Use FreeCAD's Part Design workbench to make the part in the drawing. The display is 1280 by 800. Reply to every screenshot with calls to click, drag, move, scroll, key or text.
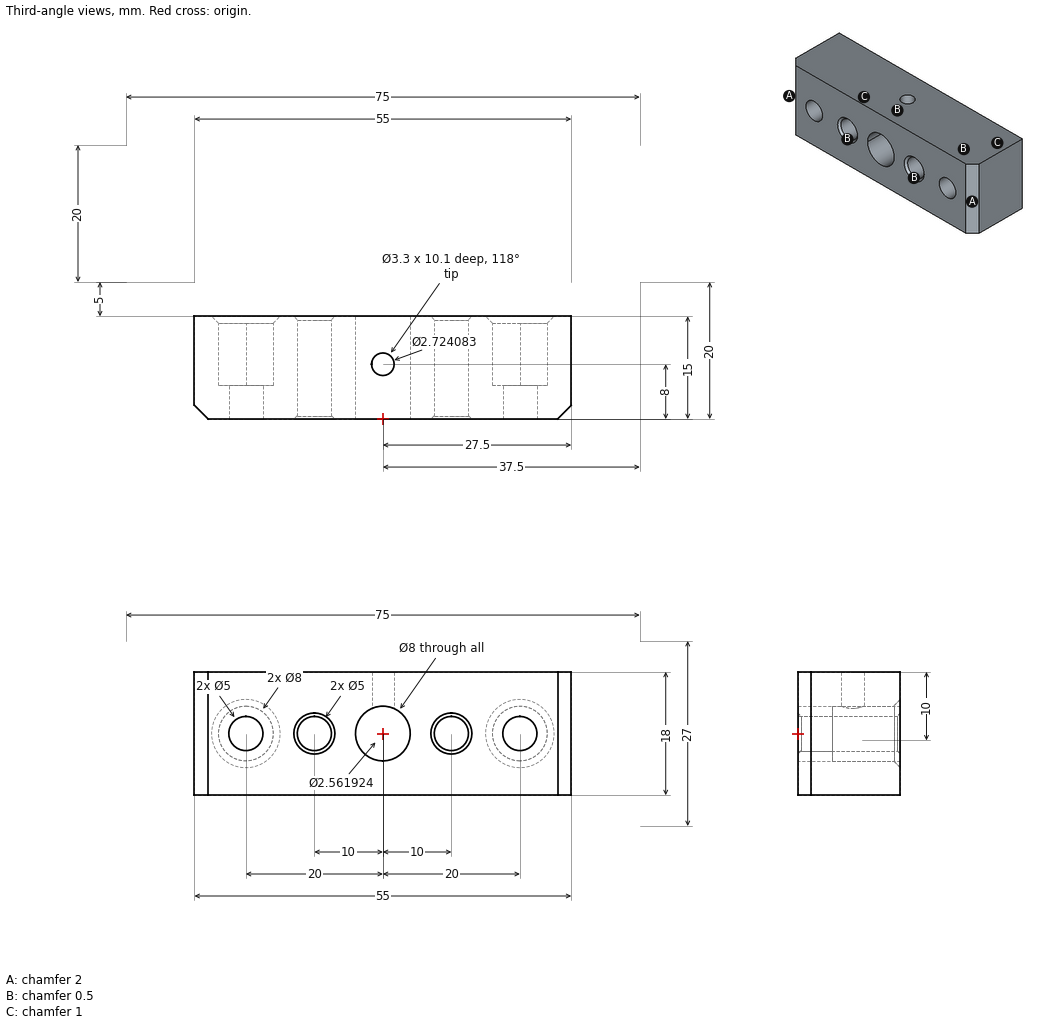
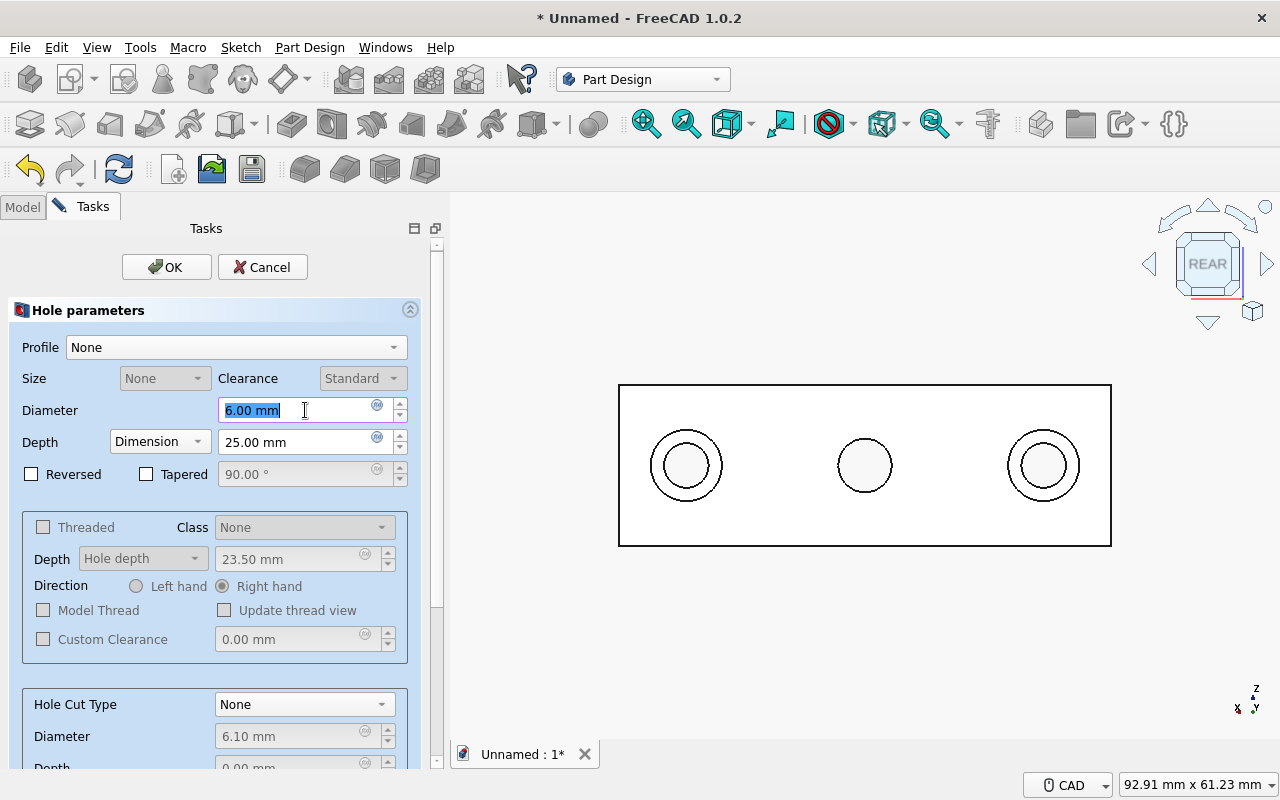
text(8)
key(Tab)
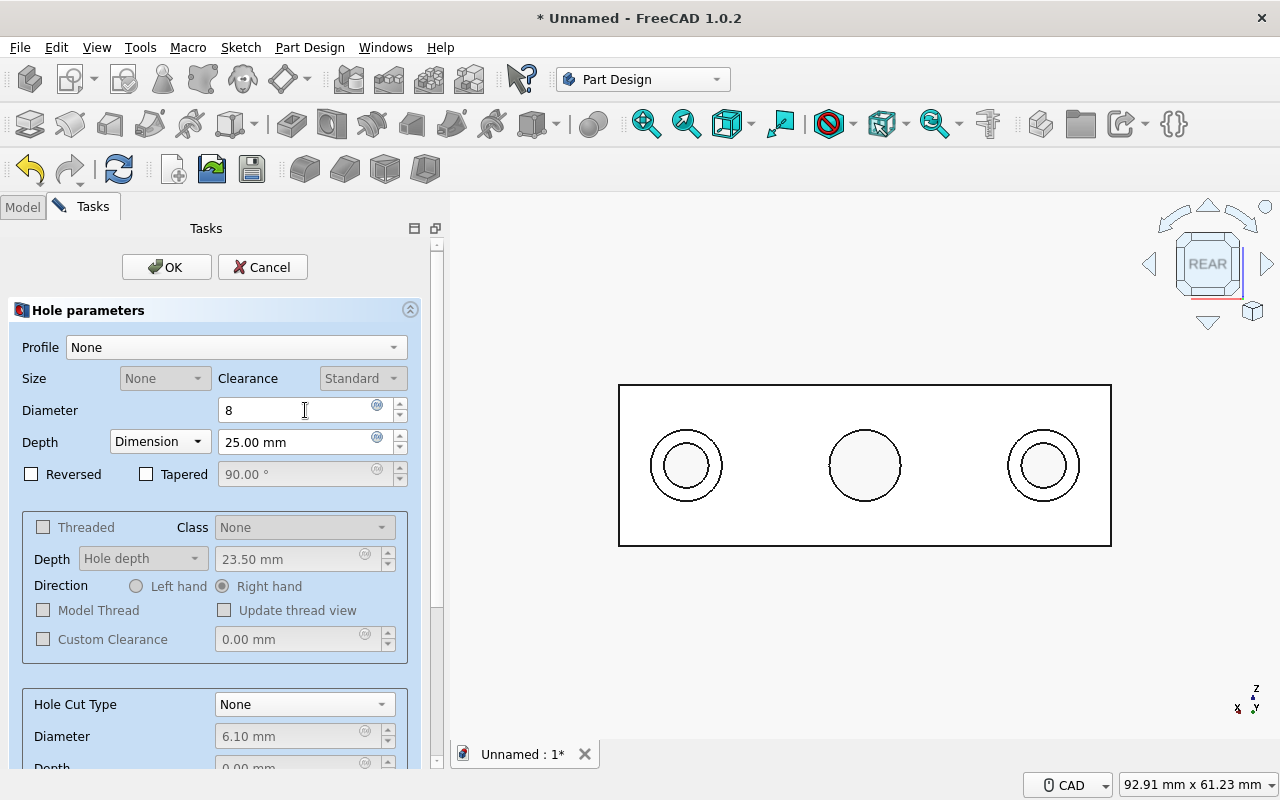
click(161, 442)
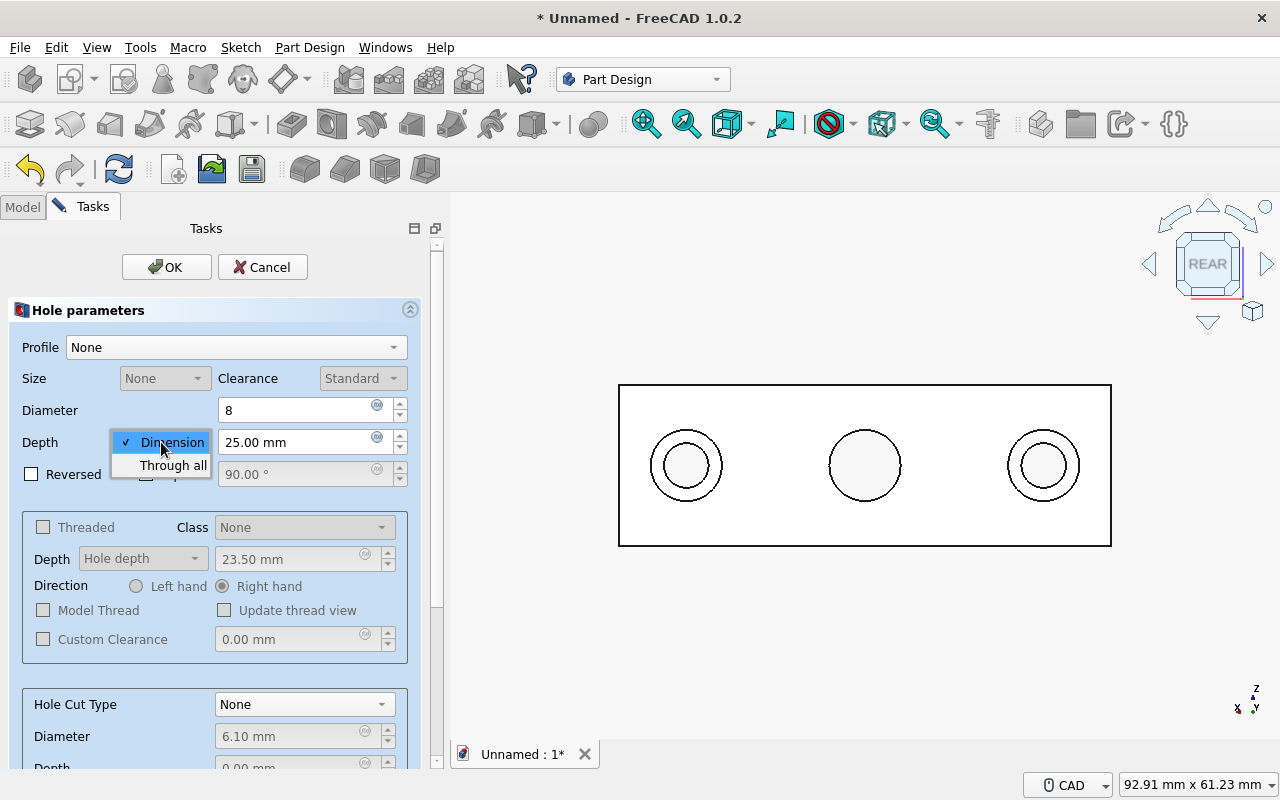
click(160, 466)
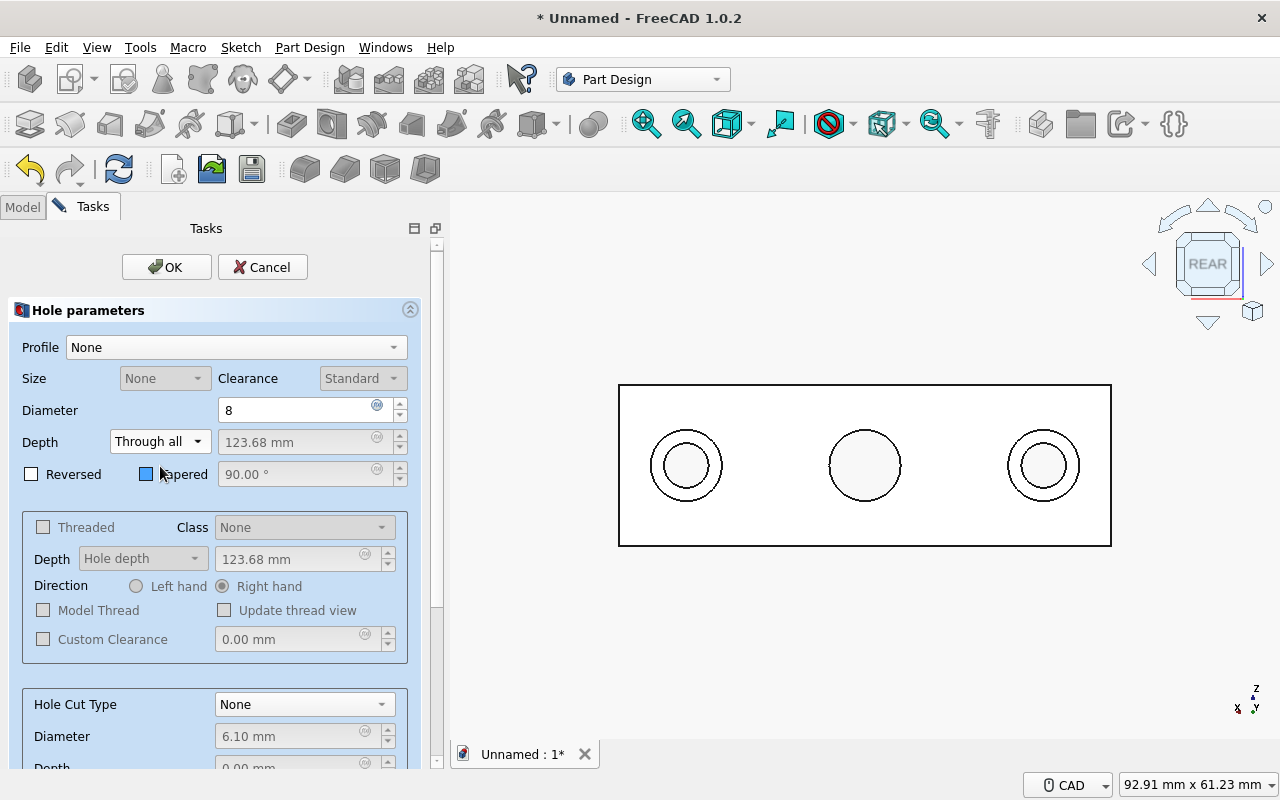
click(167, 267)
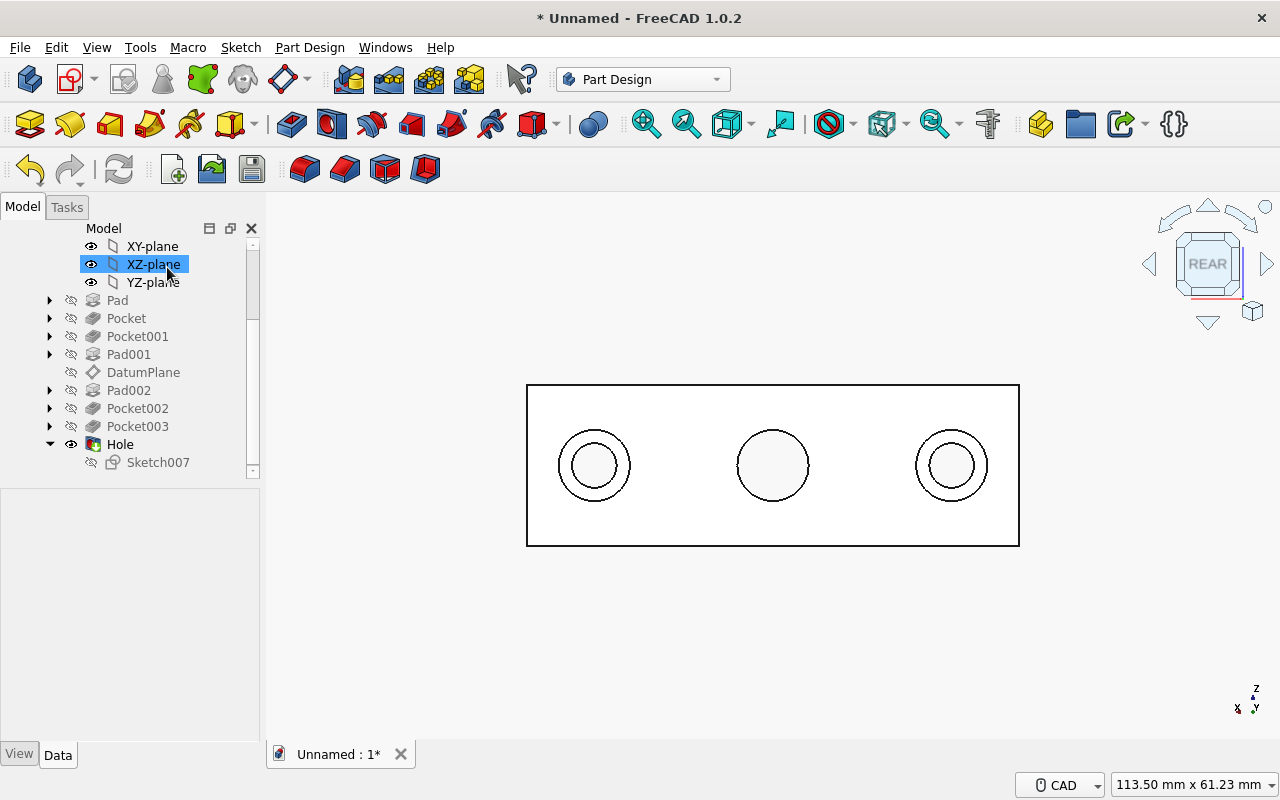
key(0)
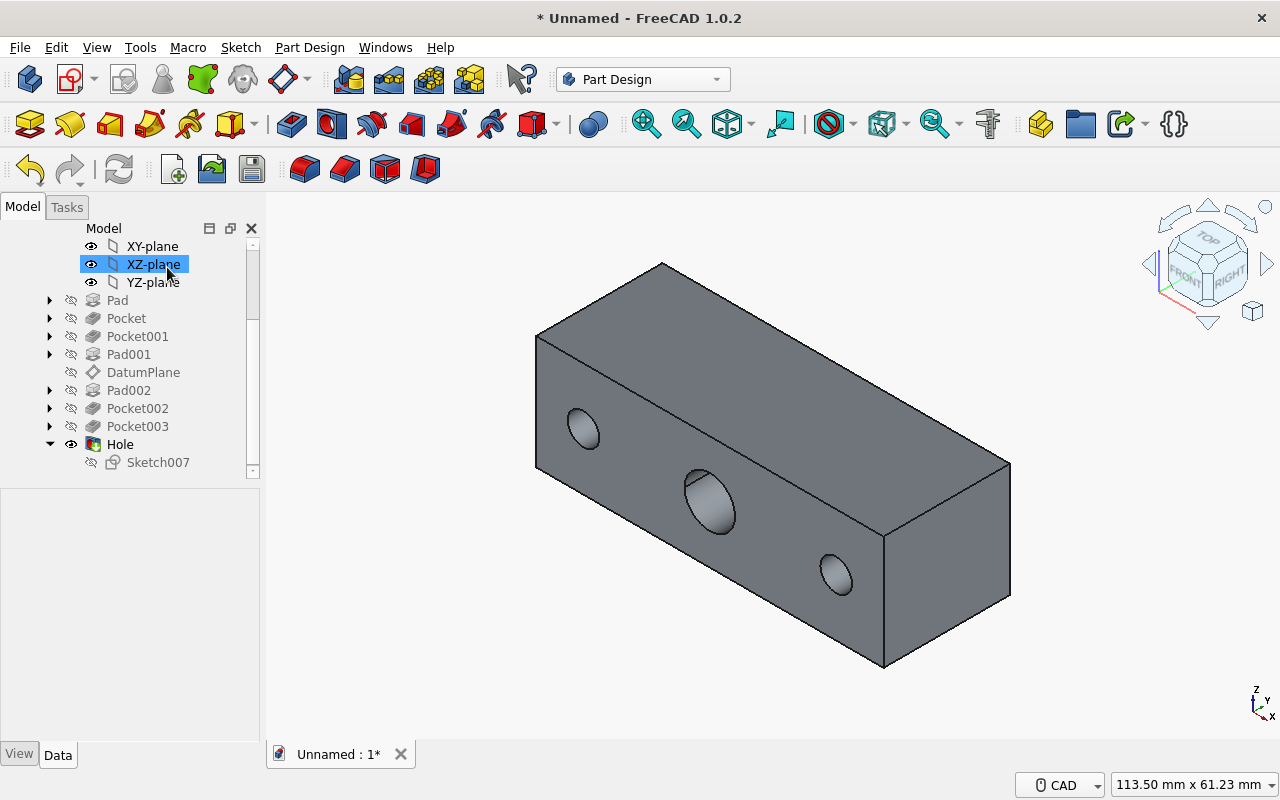
click(884, 601)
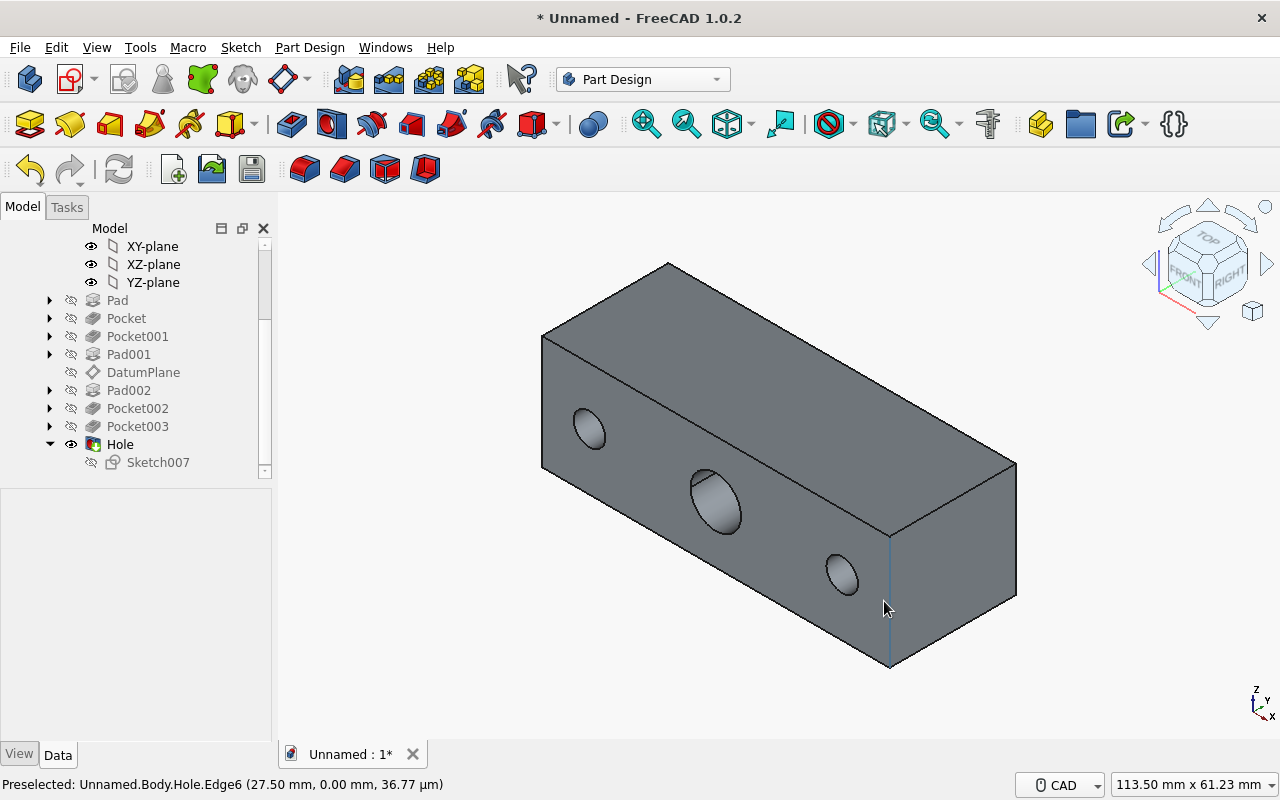
key(2)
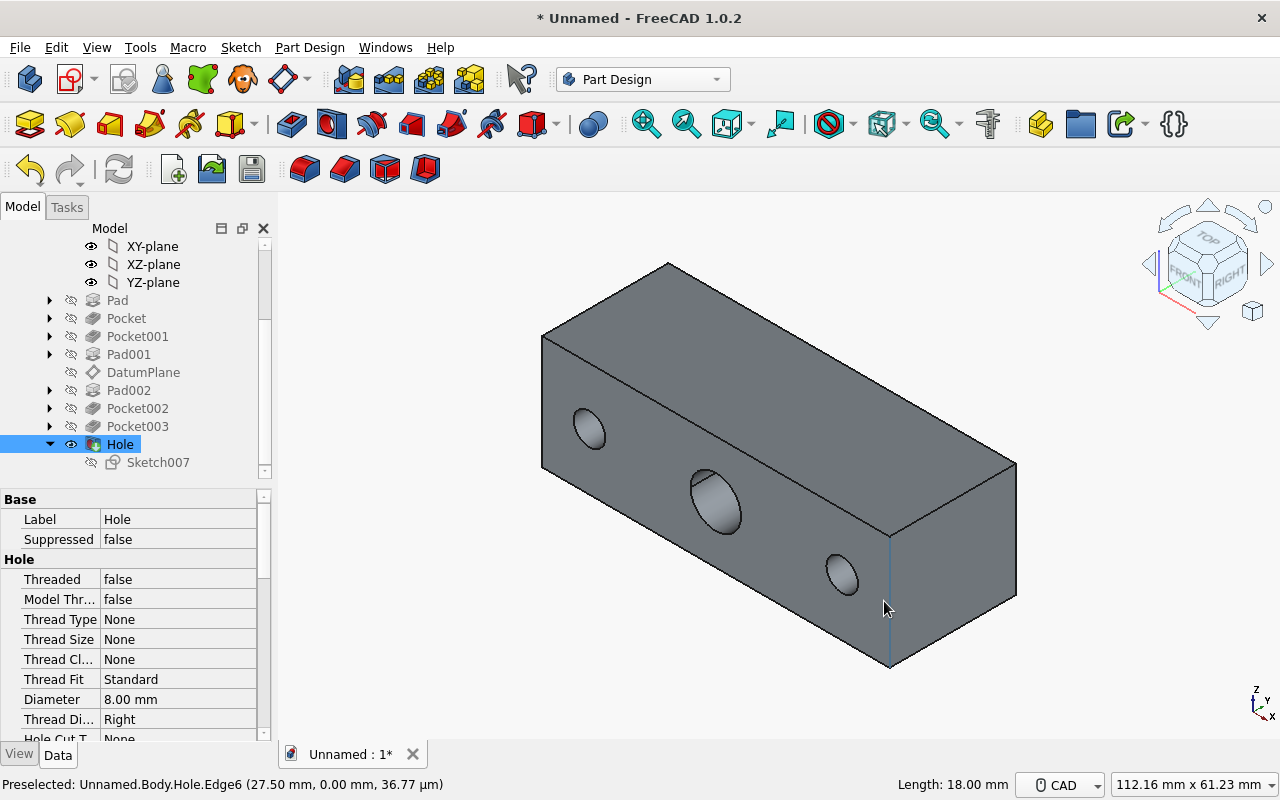
key(1)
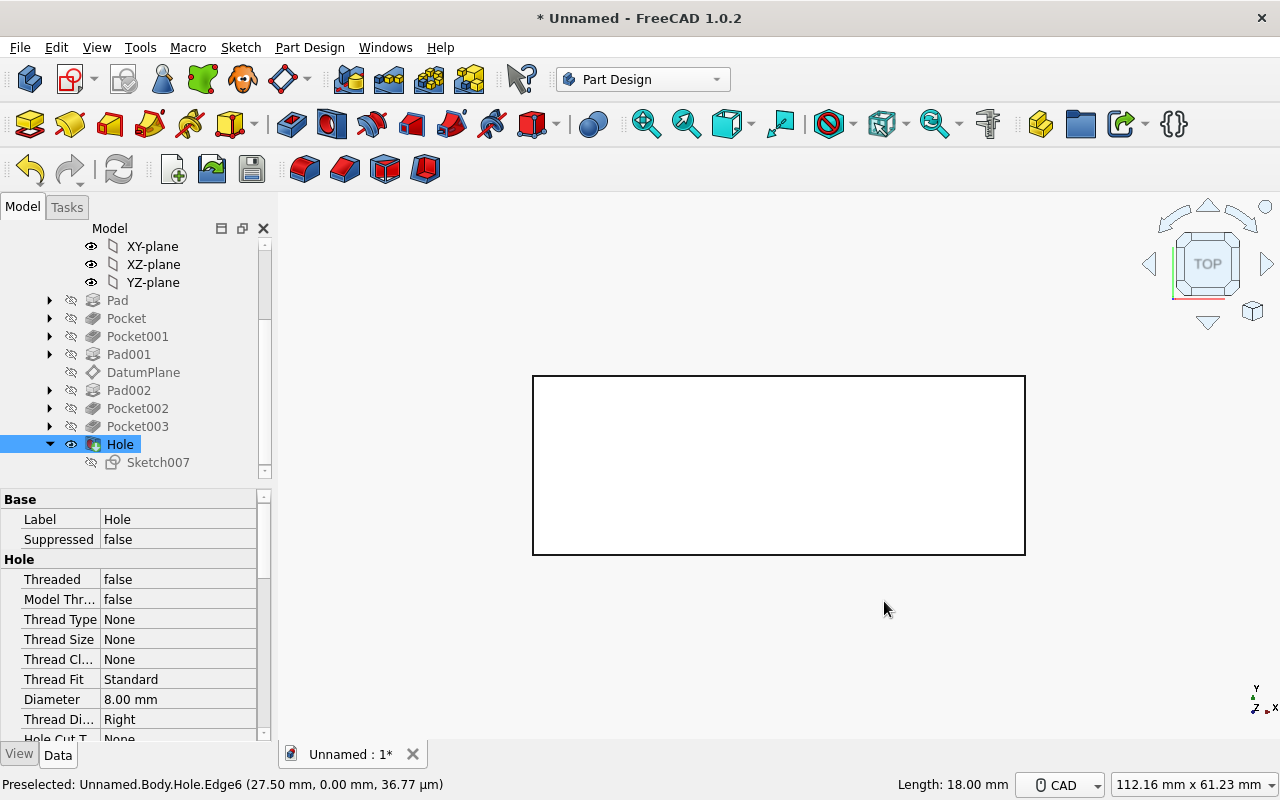
click(533, 465, ctrl)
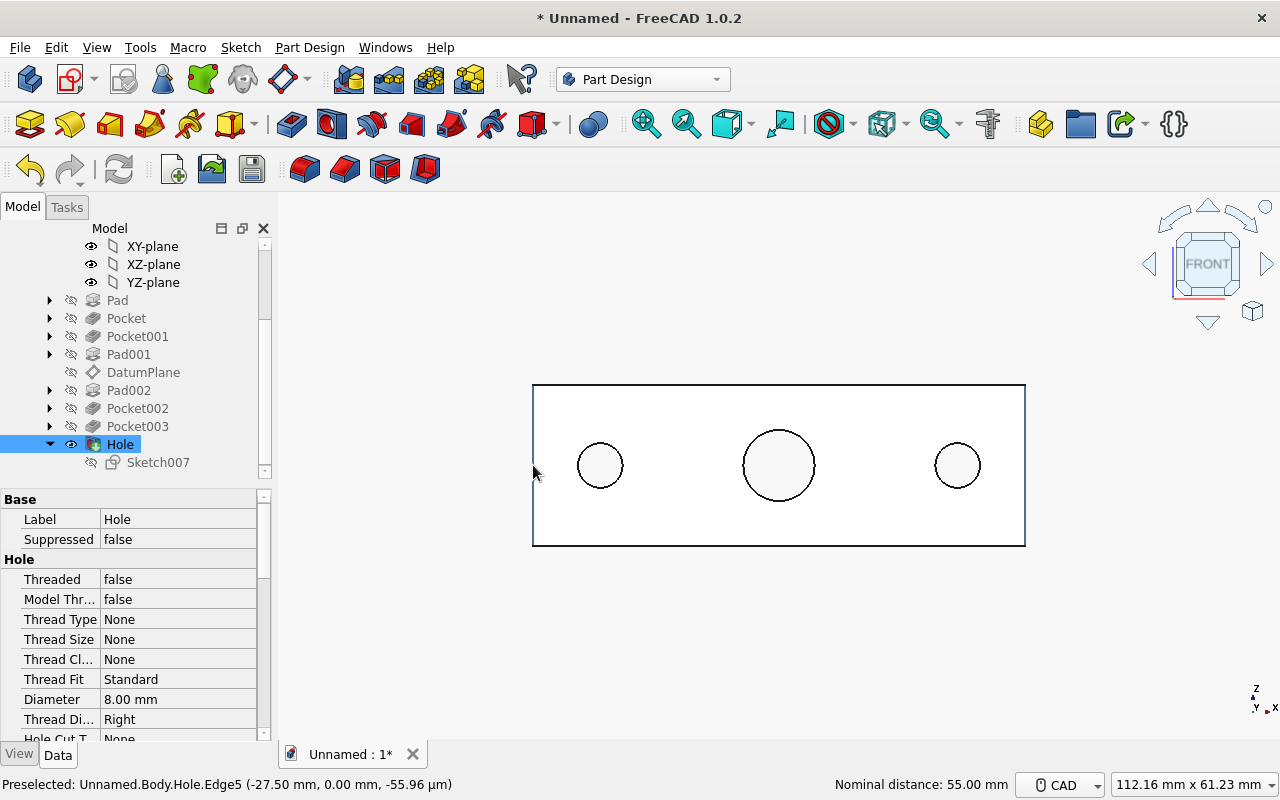
click(346, 170)